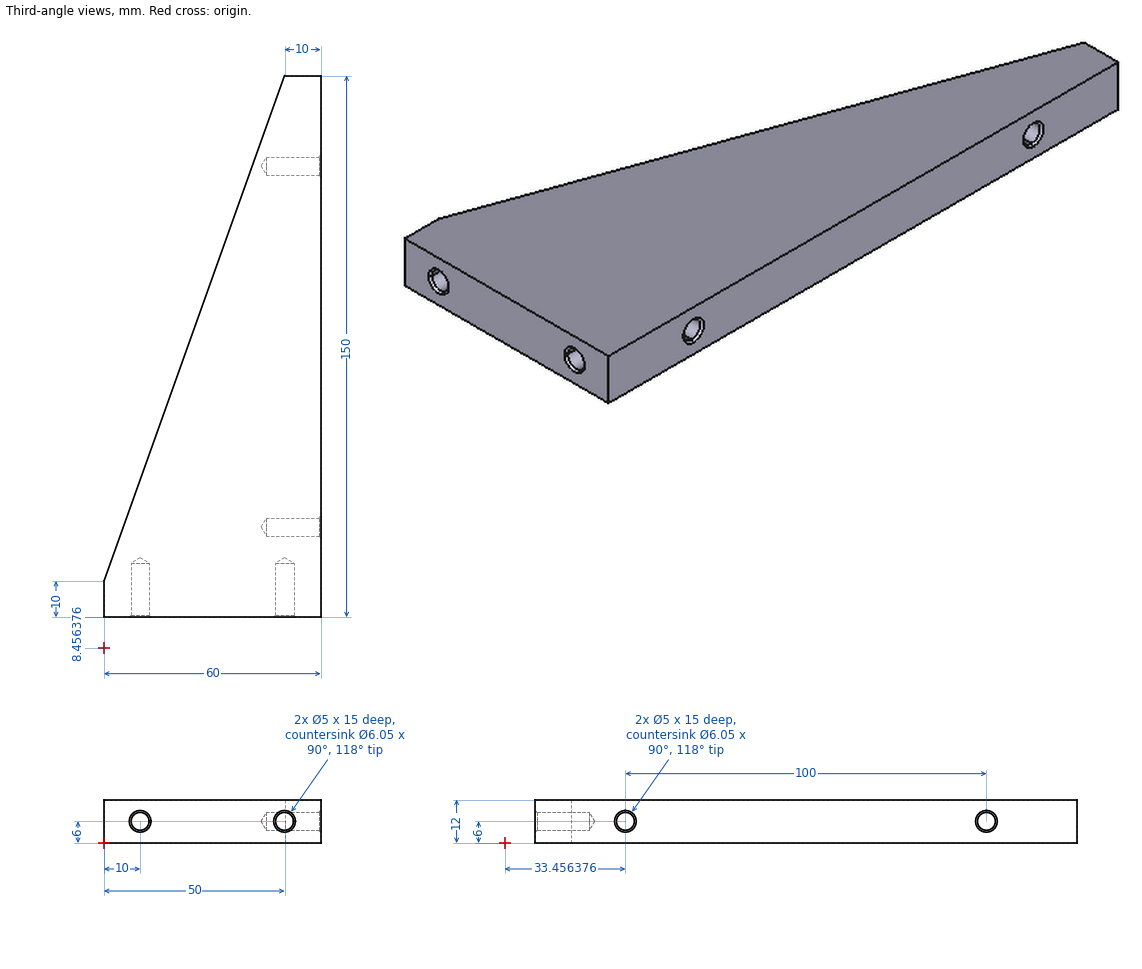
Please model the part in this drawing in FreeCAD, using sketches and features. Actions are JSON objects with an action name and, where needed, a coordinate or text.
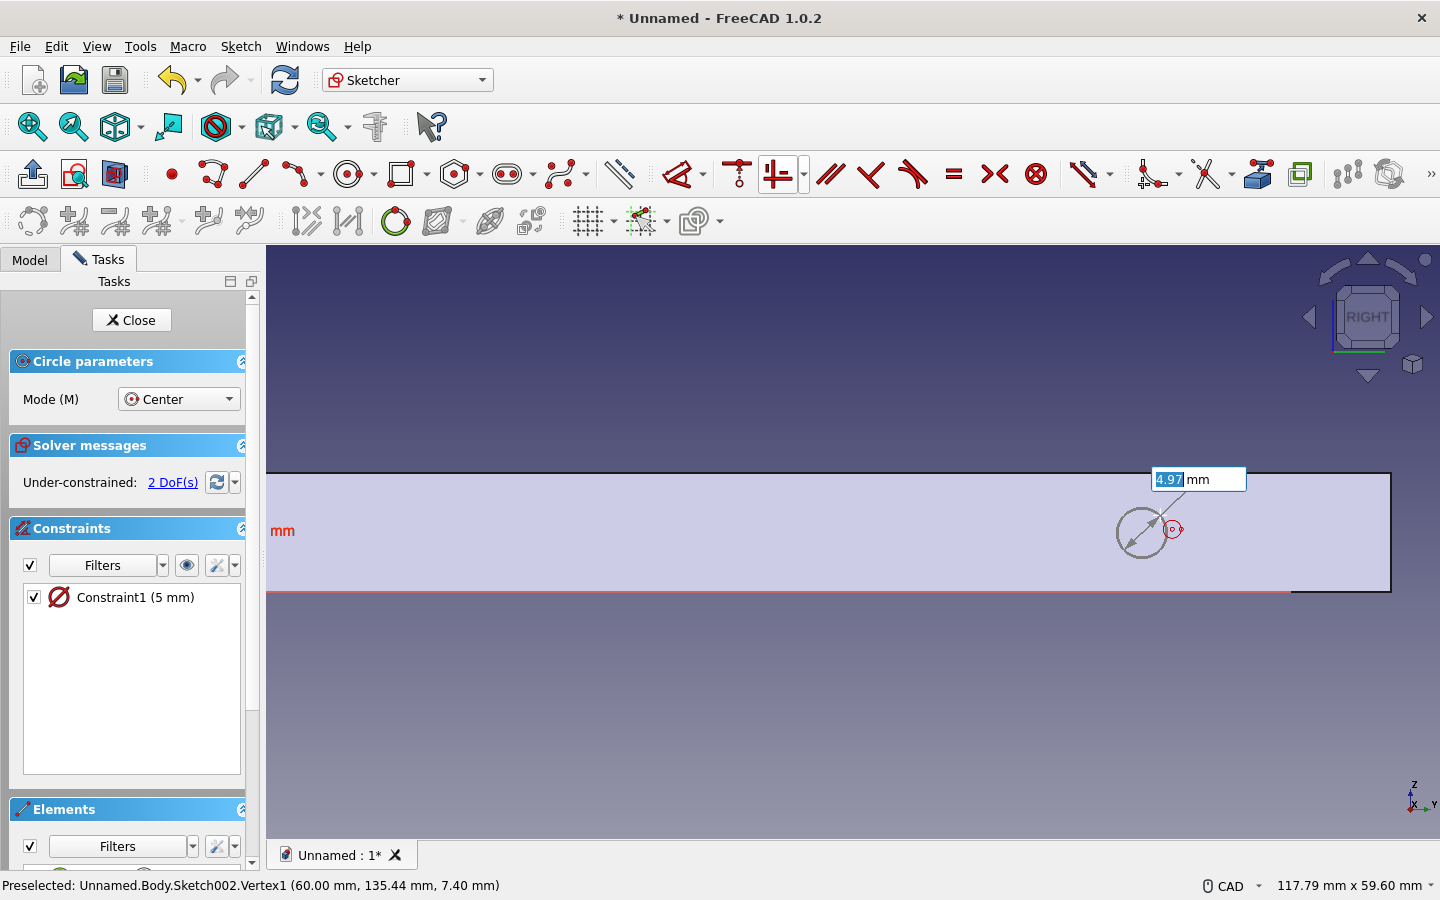
{"action": "type", "text": "5"}
{"action": "key", "text": "Return"}
{"action": "key", "text": "Escape"}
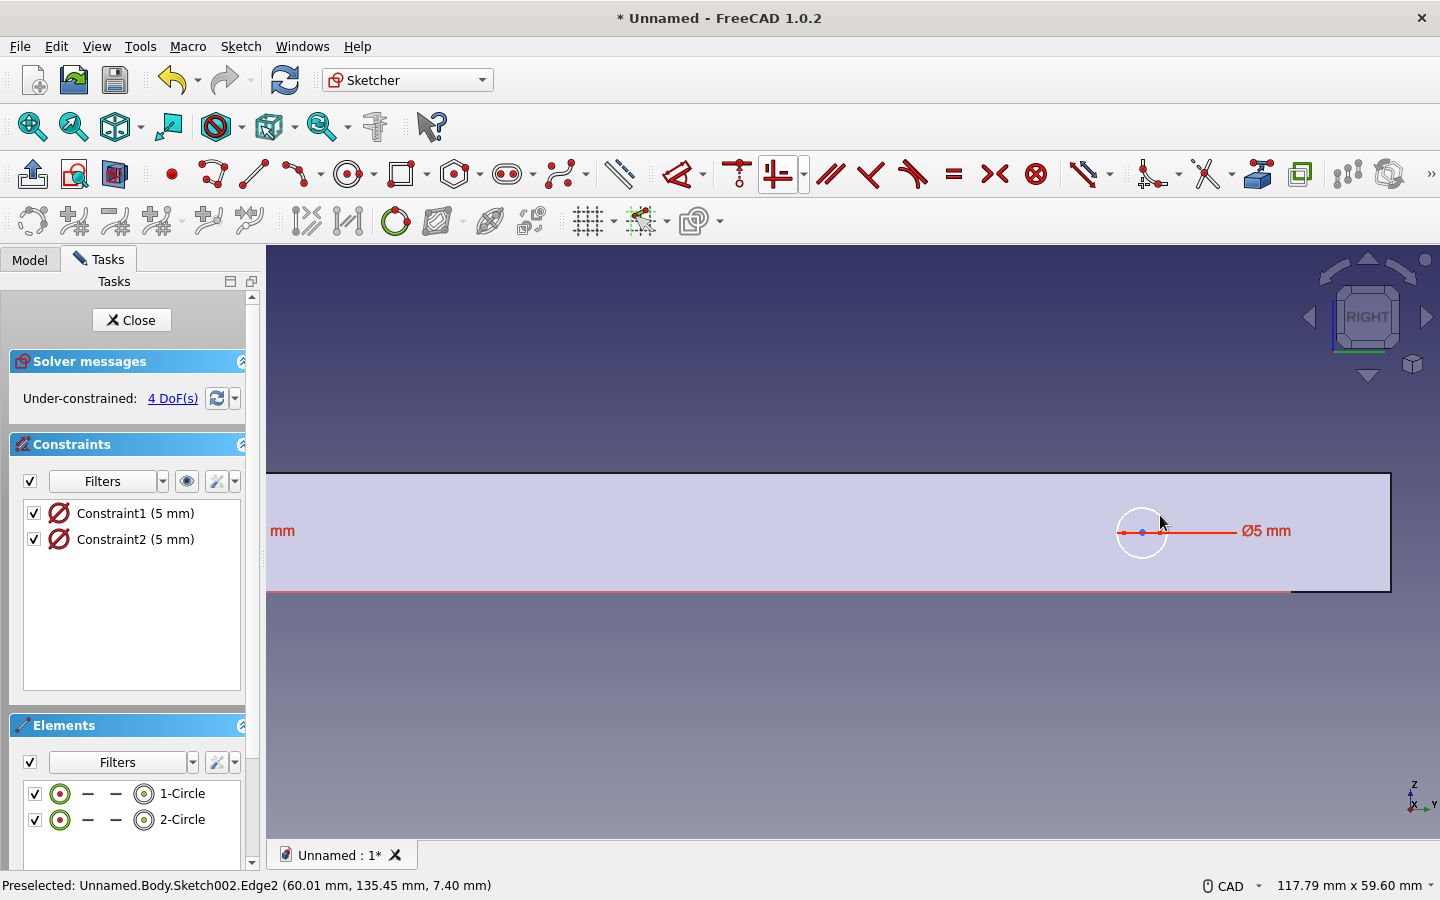
{"action": "scroll", "coordinate": [1143, 533], "scroll_direction": "down", "scroll_amount": 3}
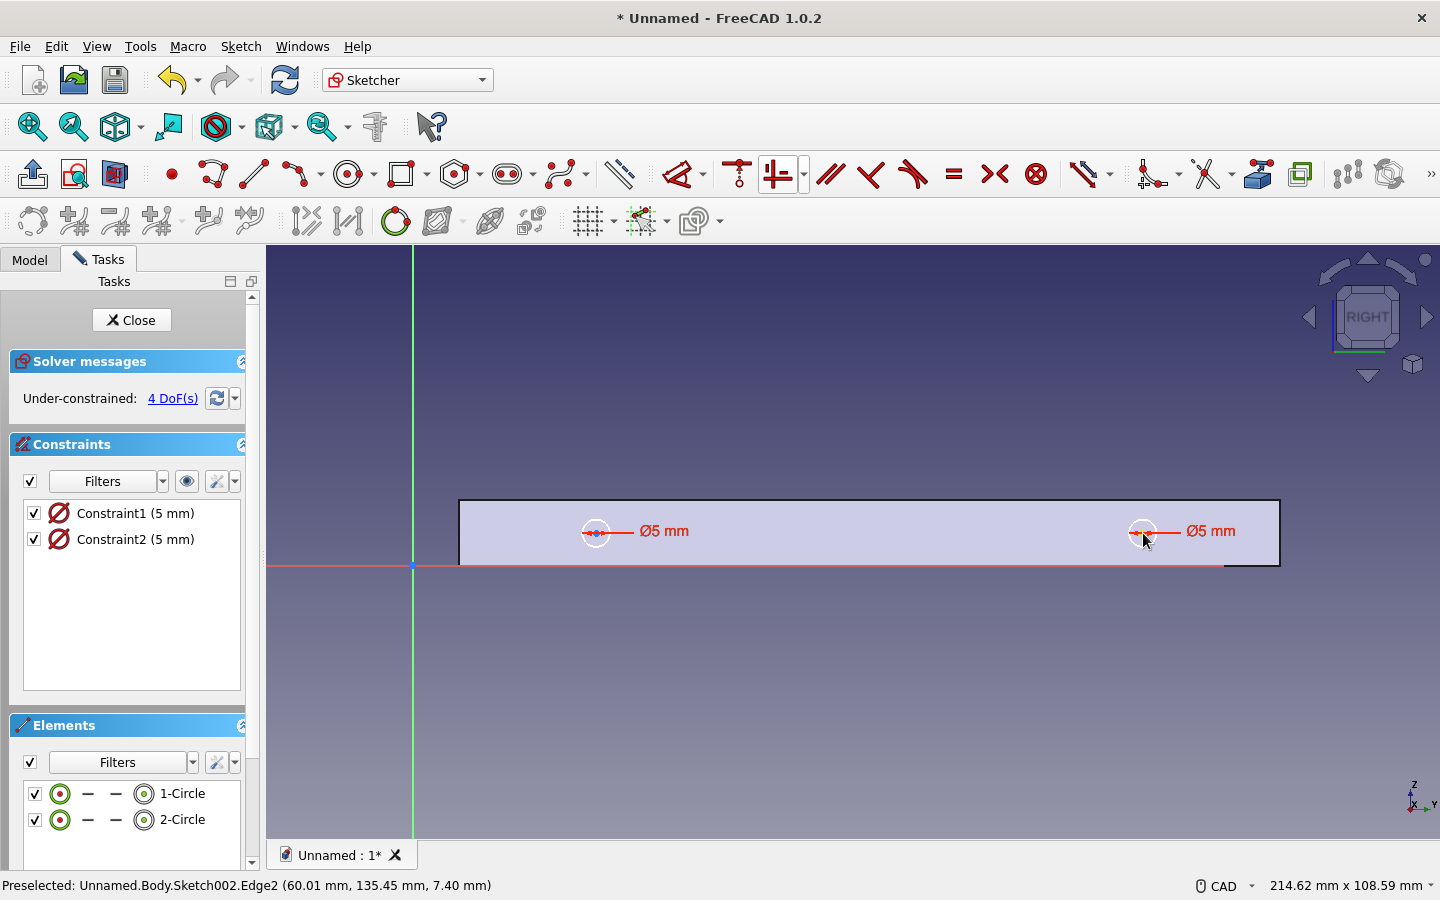
{"action": "left_click", "coordinate": [596, 533]}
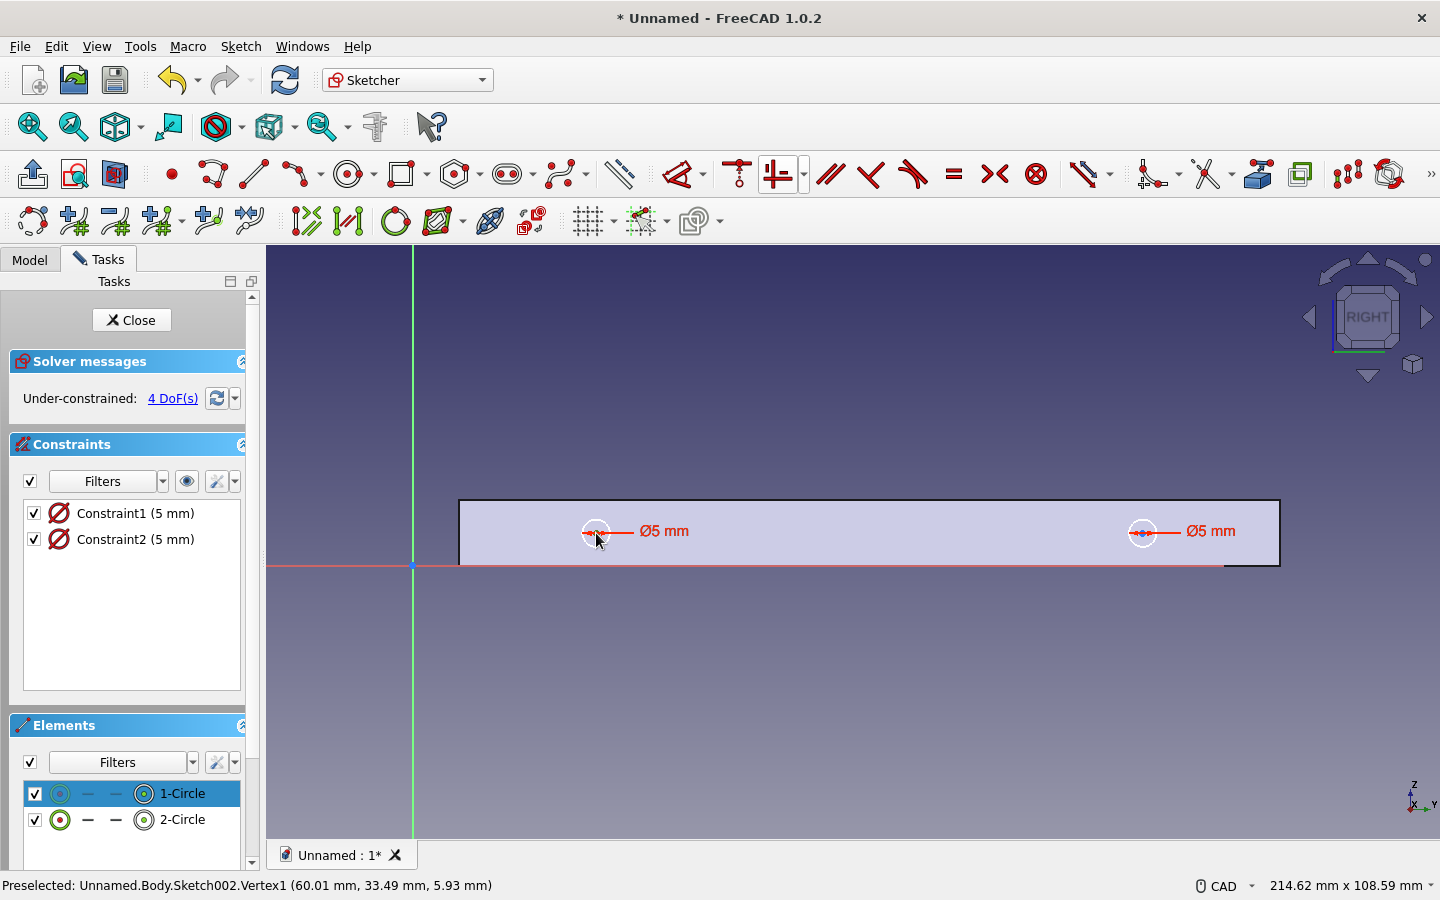
{"action": "left_click", "coordinate": [1143, 533]}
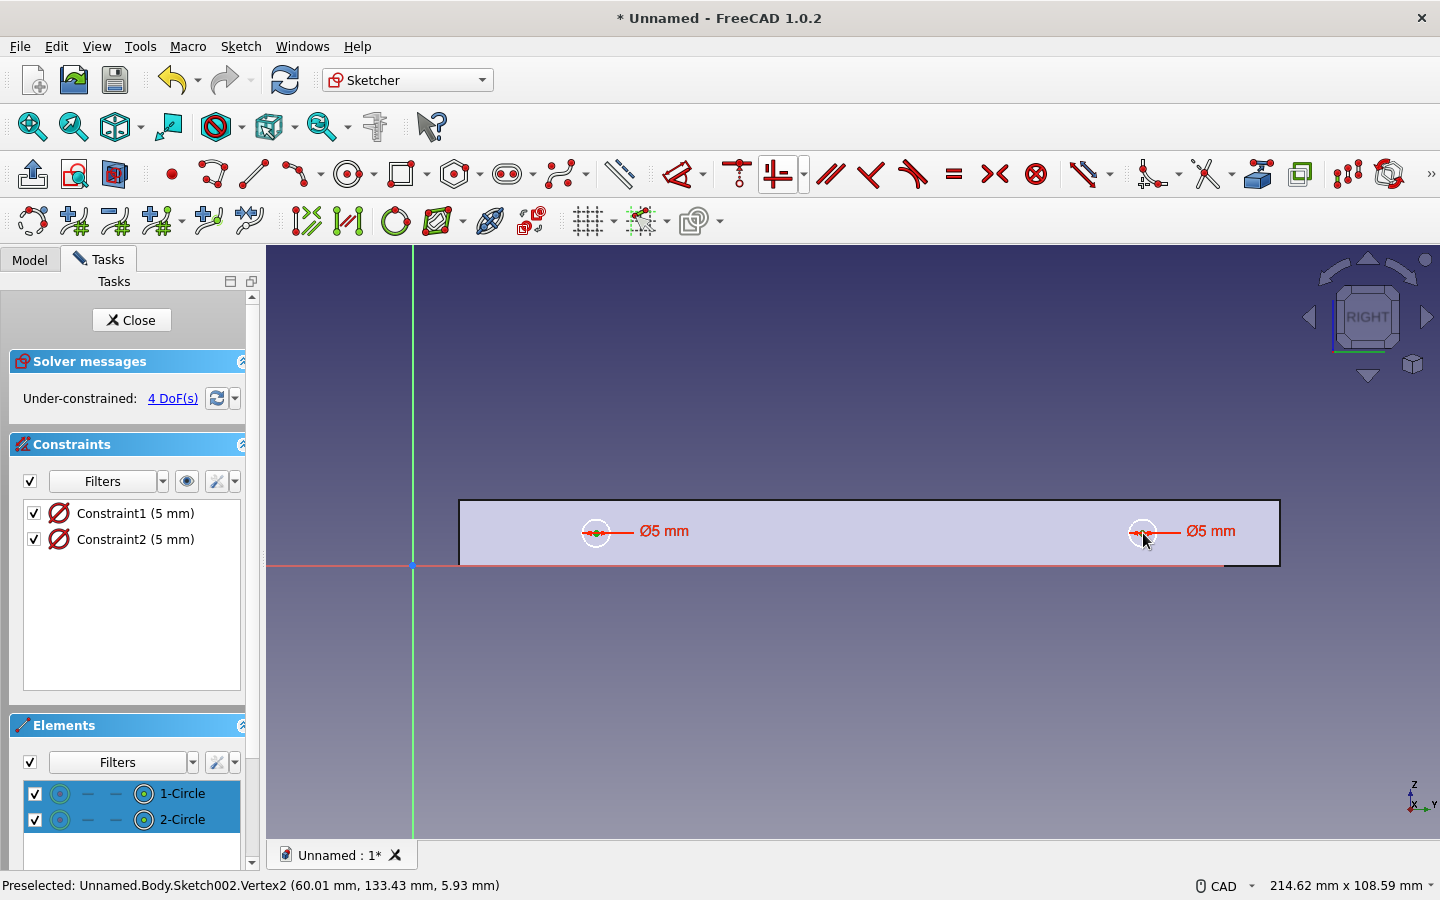
{"action": "left_click", "coordinate": [804, 174]}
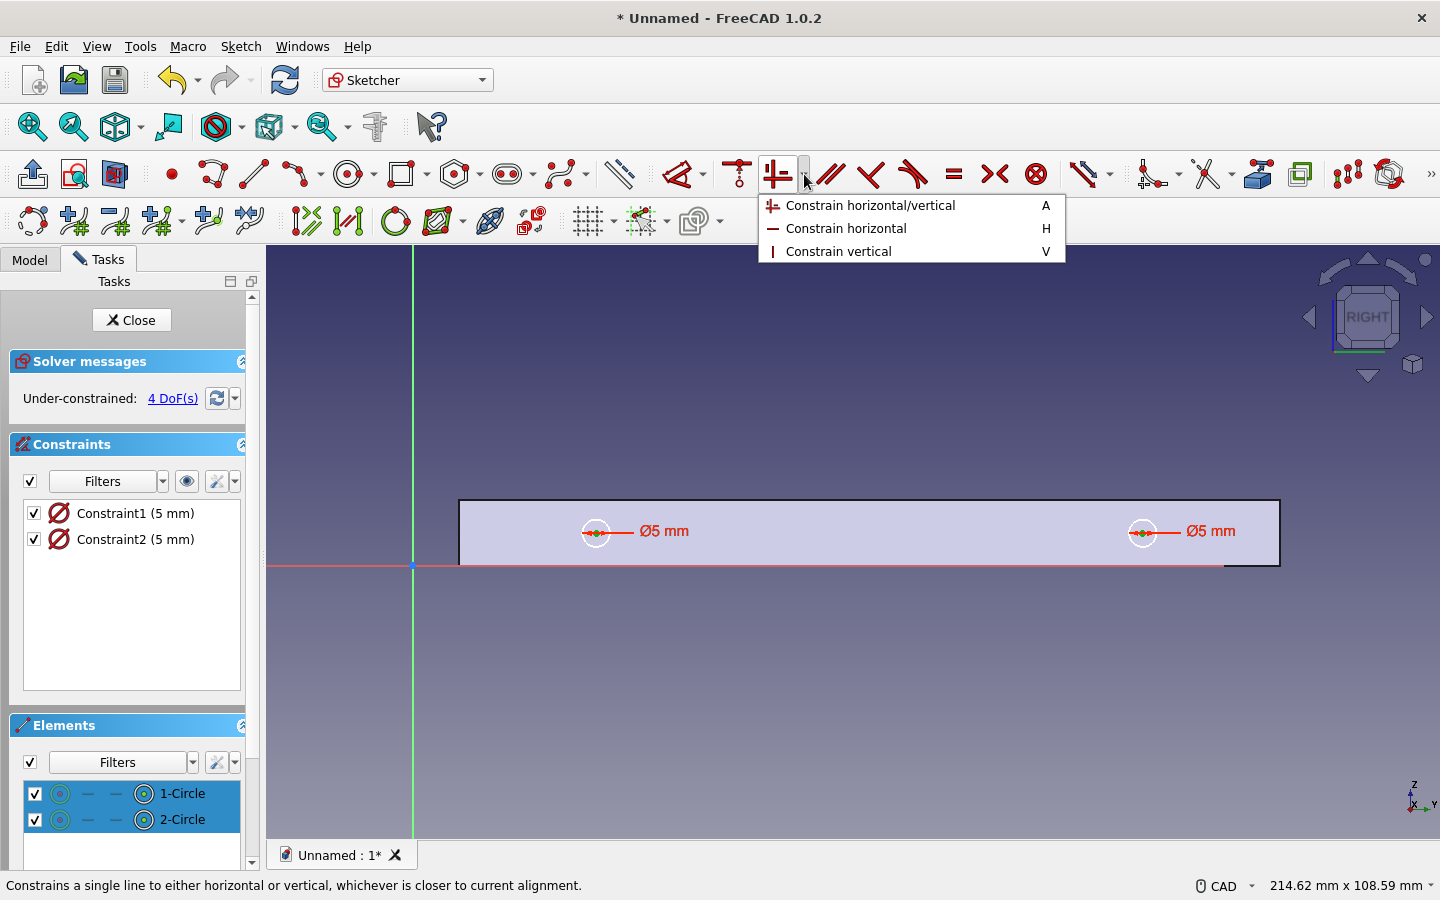
{"action": "left_click", "coordinate": [912, 228]}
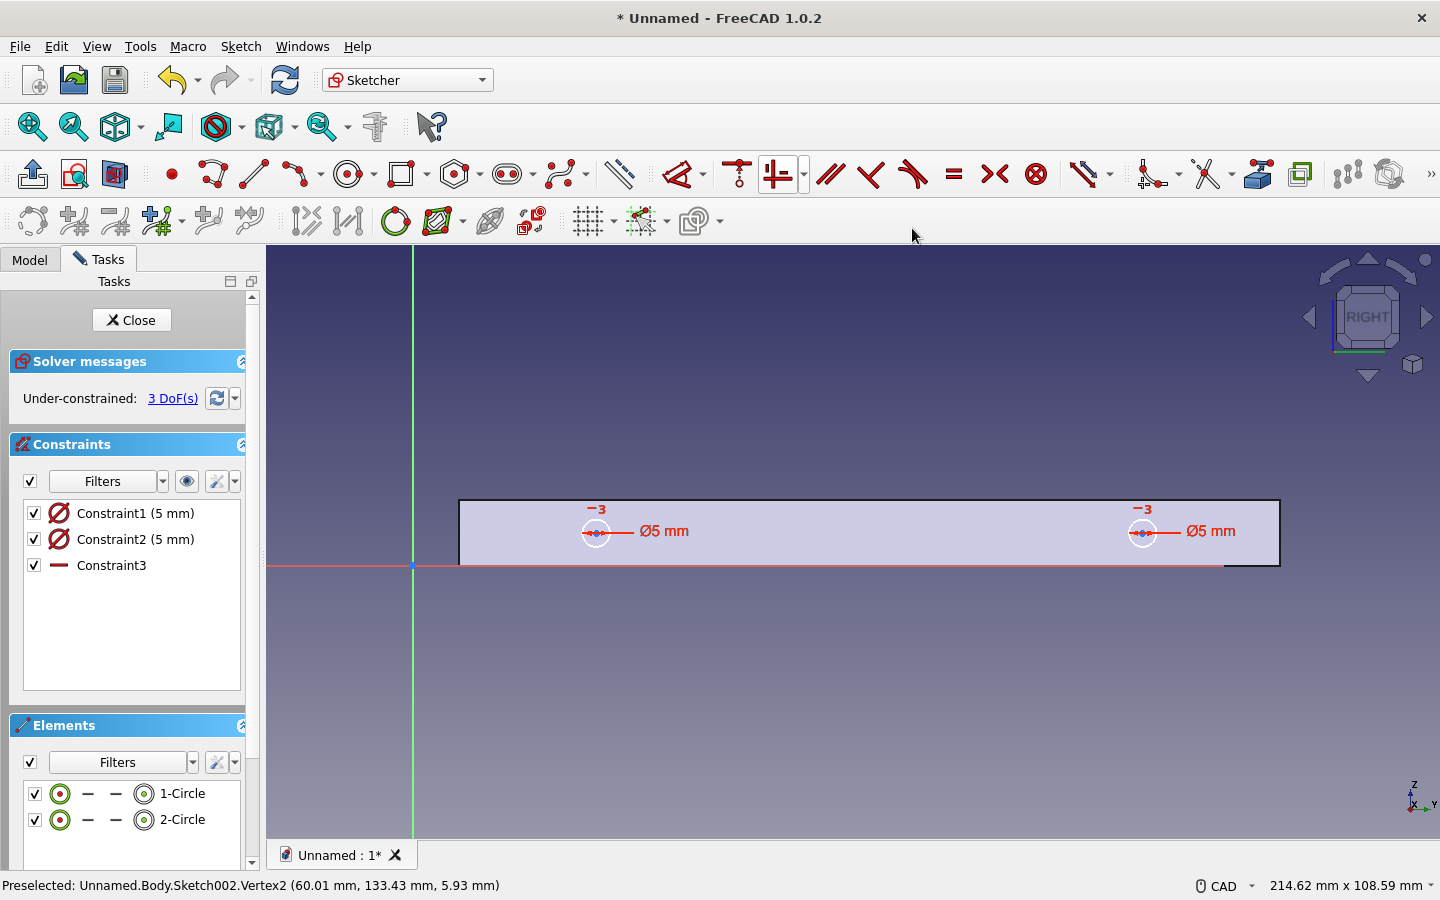
{"action": "left_click", "coordinate": [676, 174]}